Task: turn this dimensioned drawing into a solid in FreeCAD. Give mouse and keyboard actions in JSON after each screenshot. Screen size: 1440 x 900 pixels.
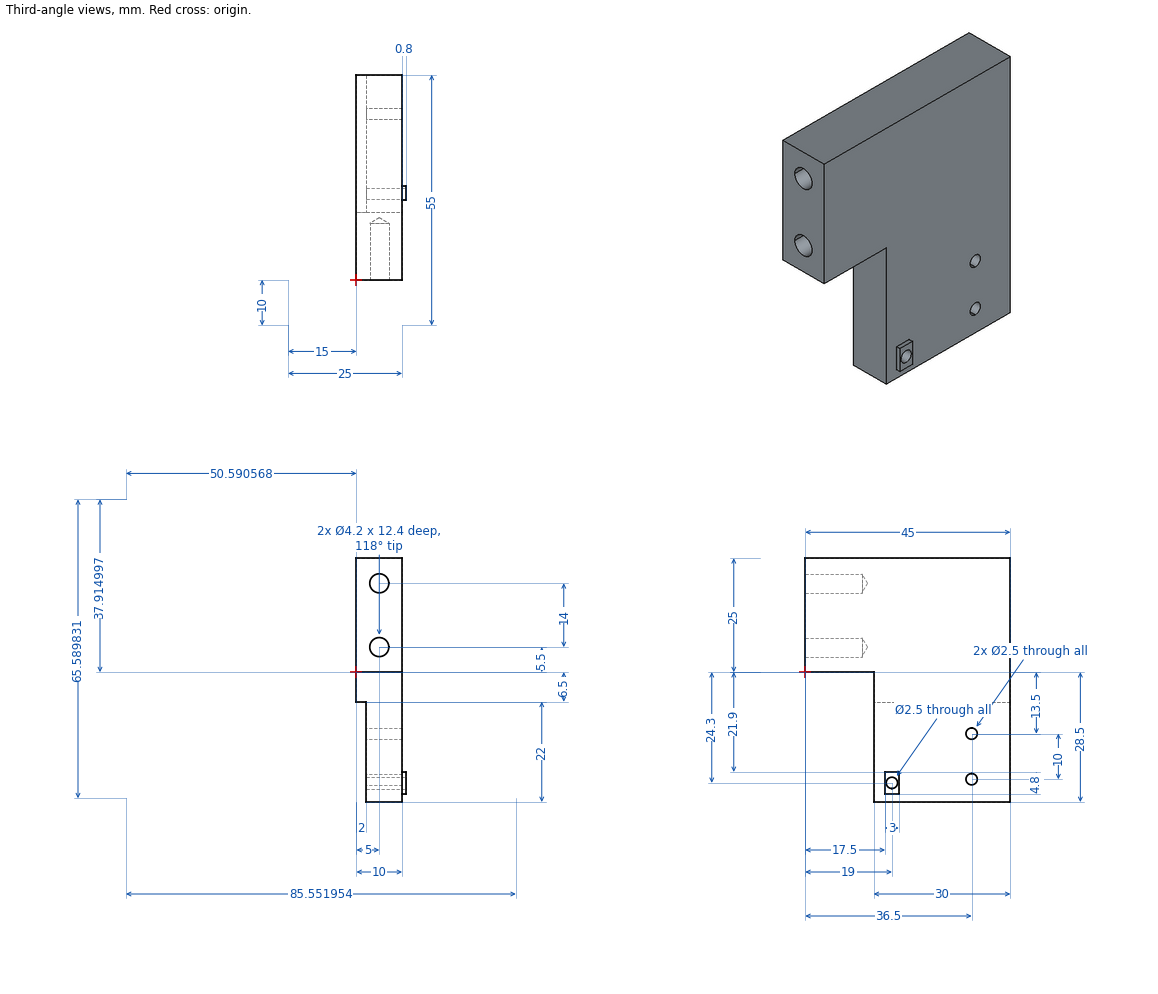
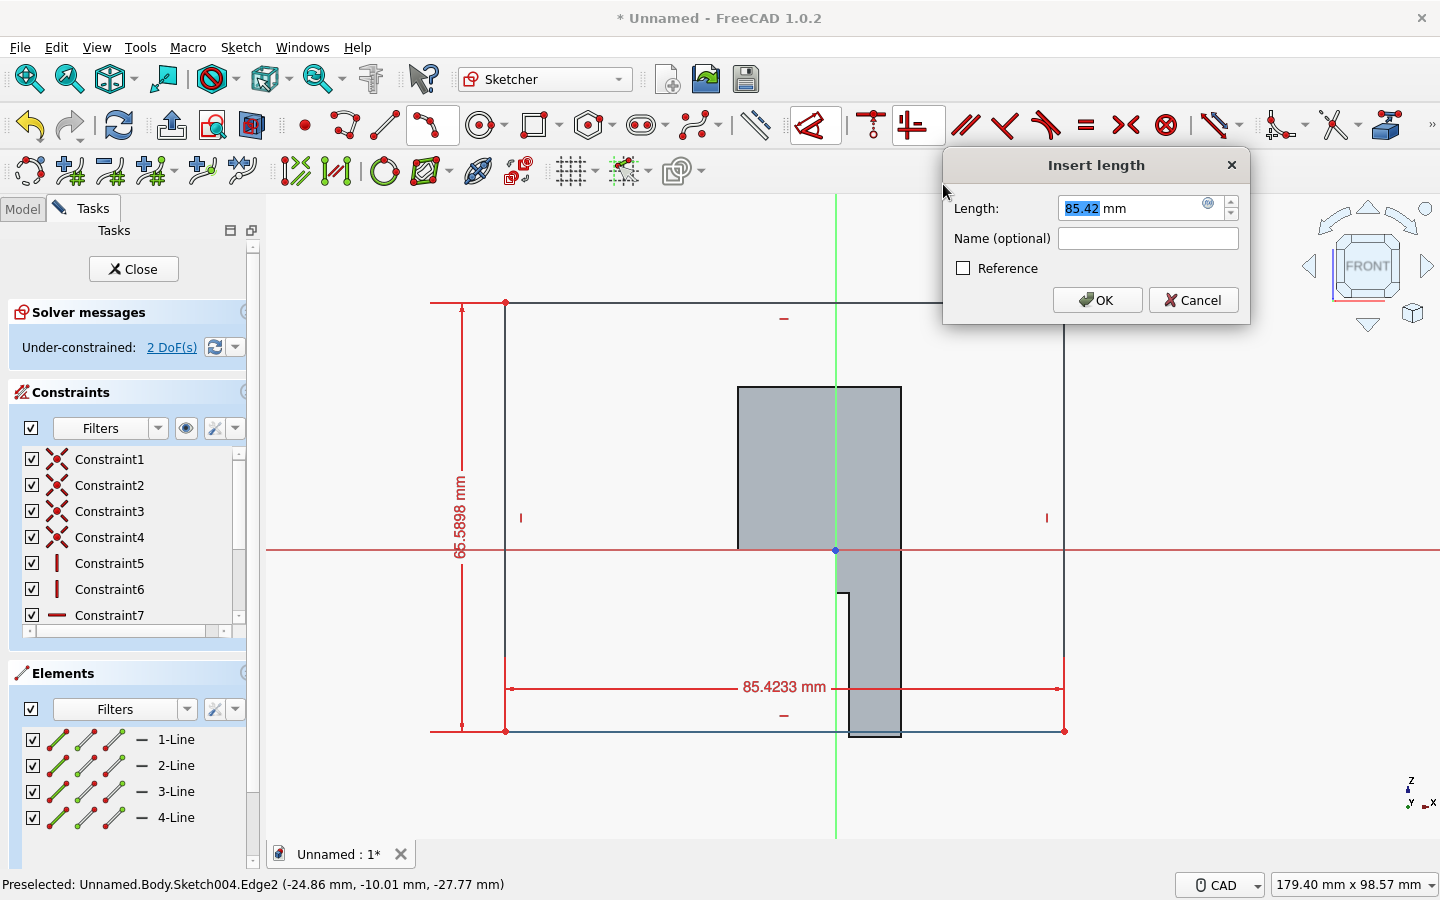
{"action": "type", "text": "85.551954"}
{"action": "key", "text": "Return"}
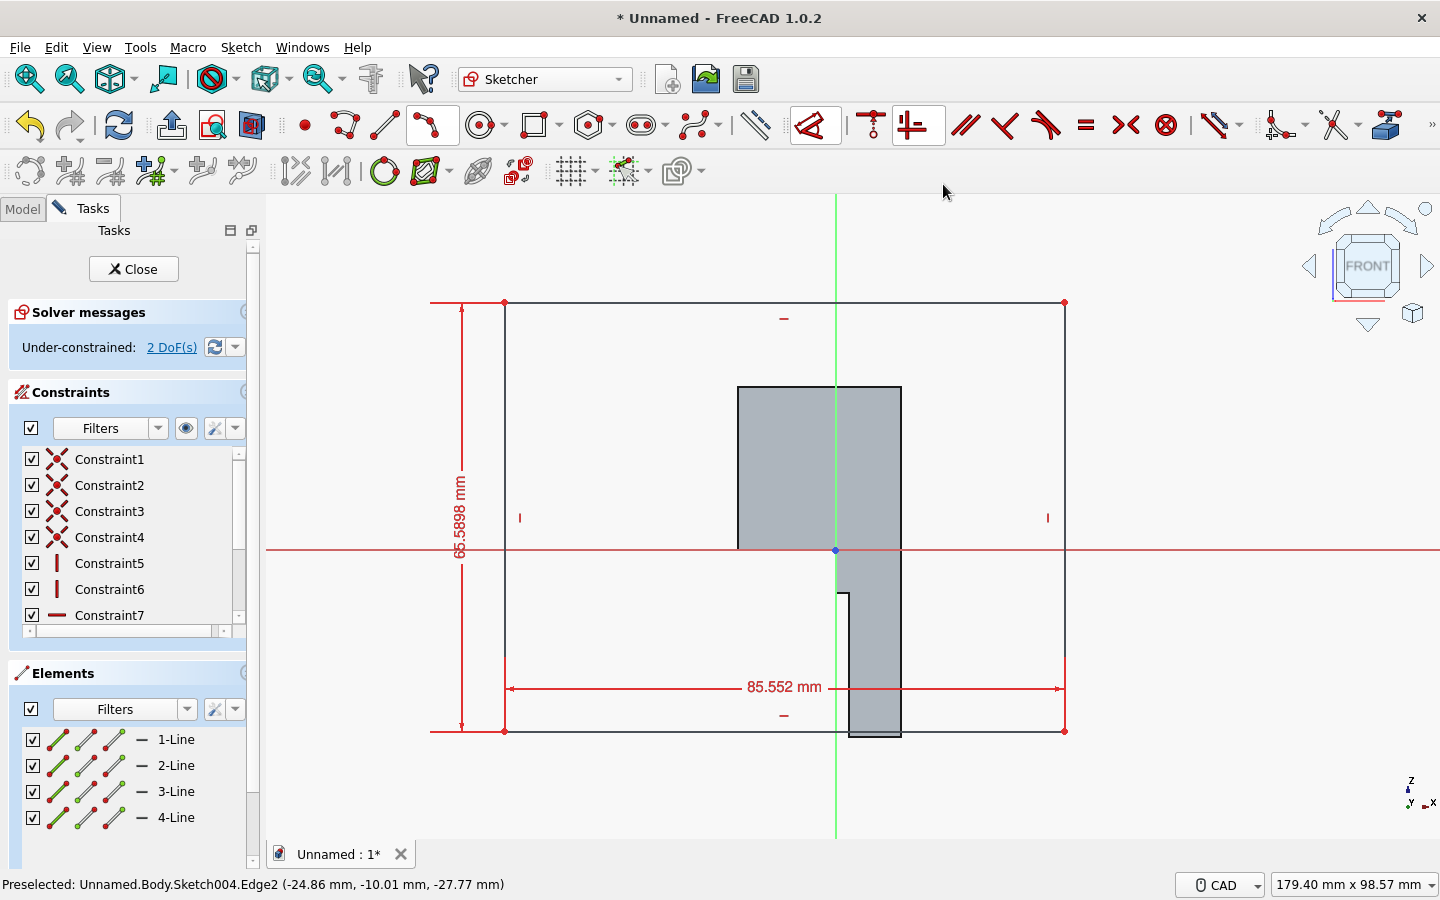
{"action": "left_click", "coordinate": [505, 303]}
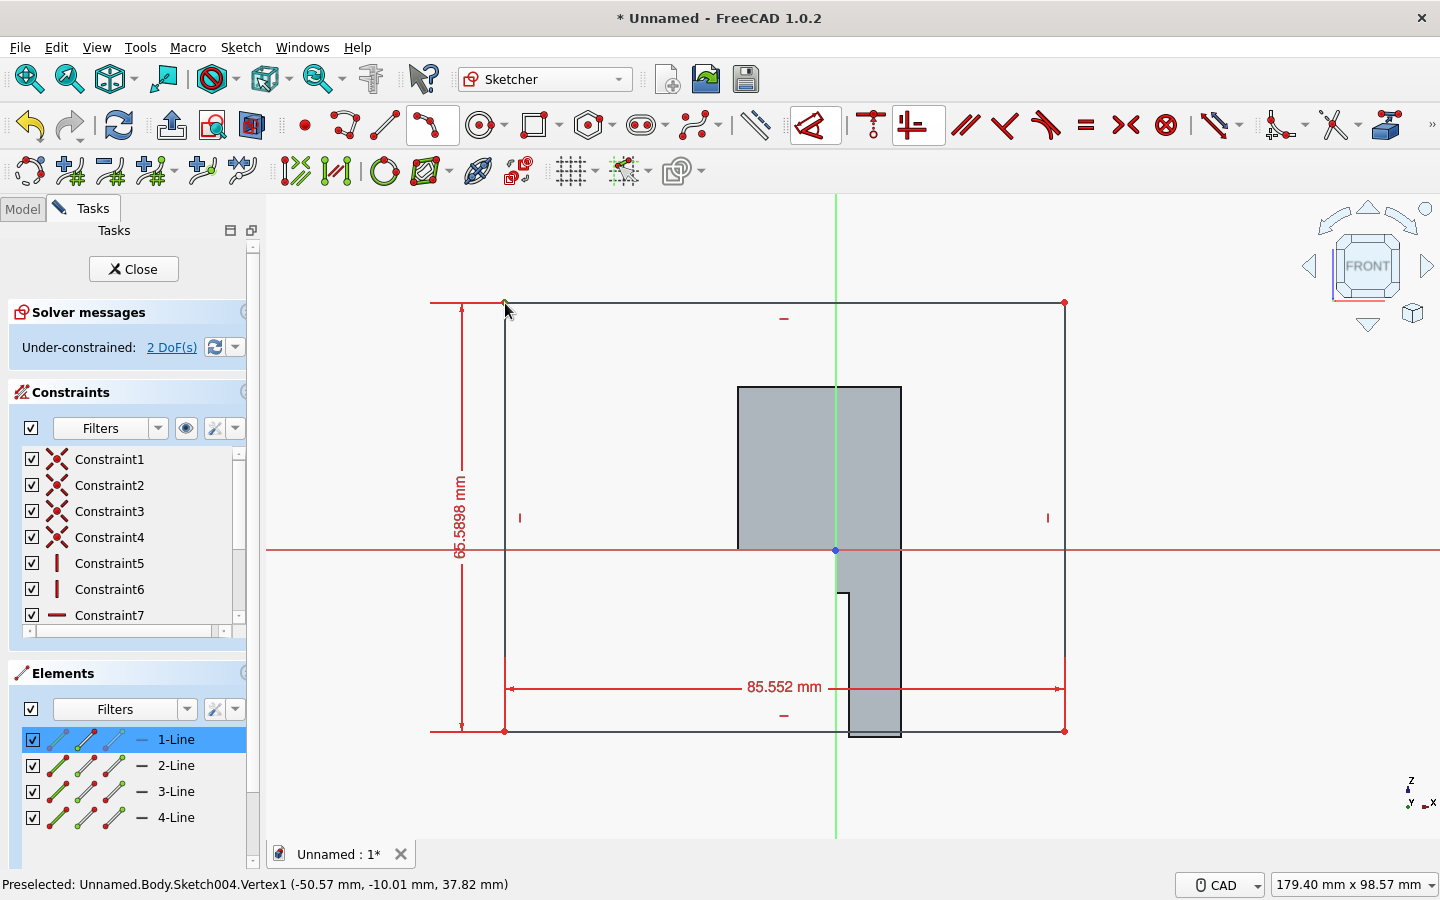
{"action": "left_click", "coordinate": [836, 126]}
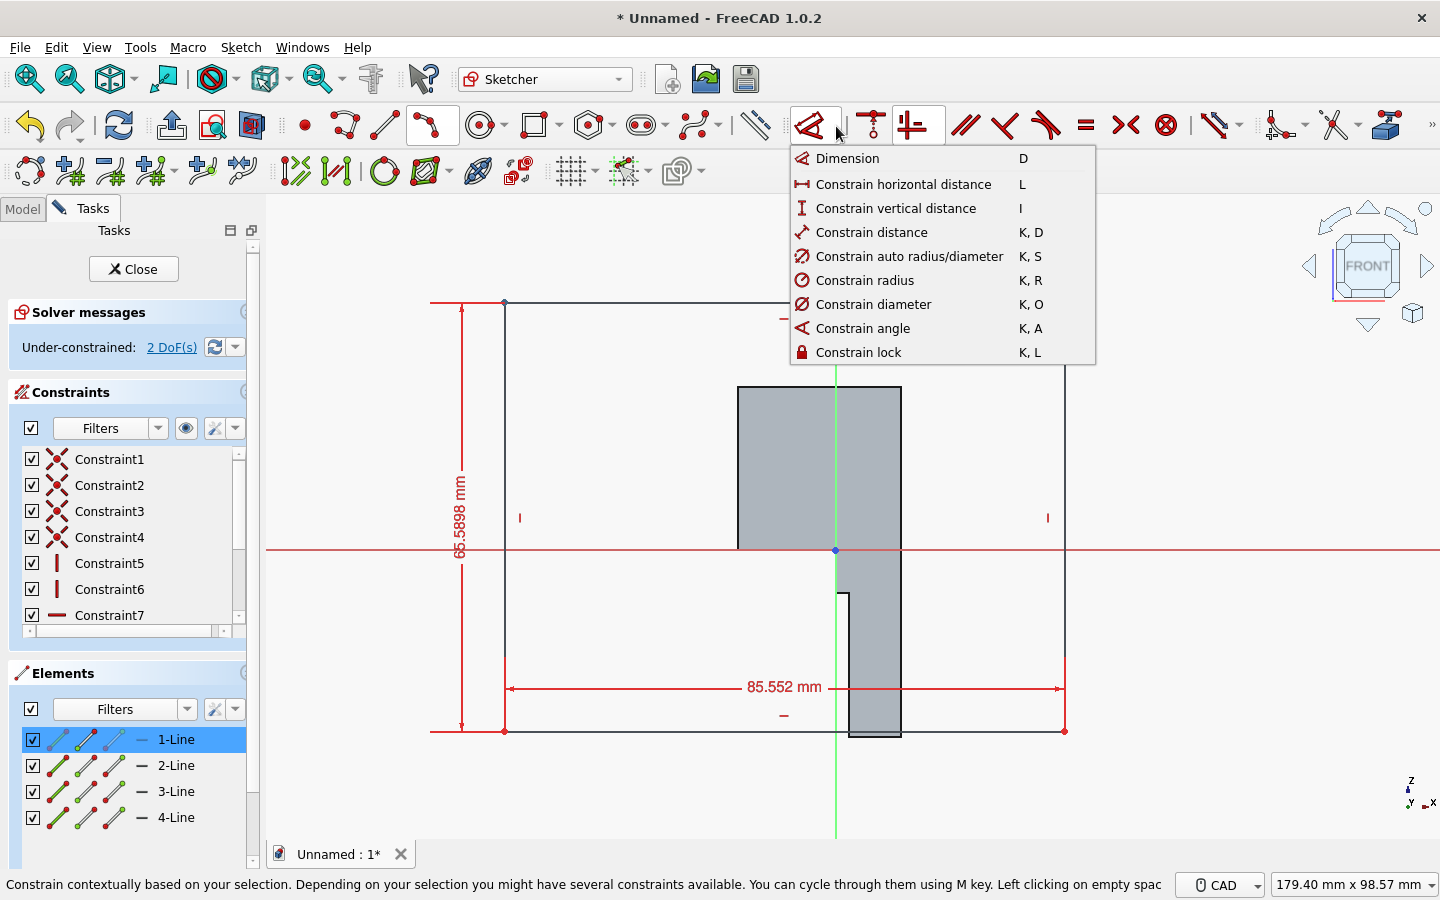
{"action": "left_click", "coordinate": [943, 184]}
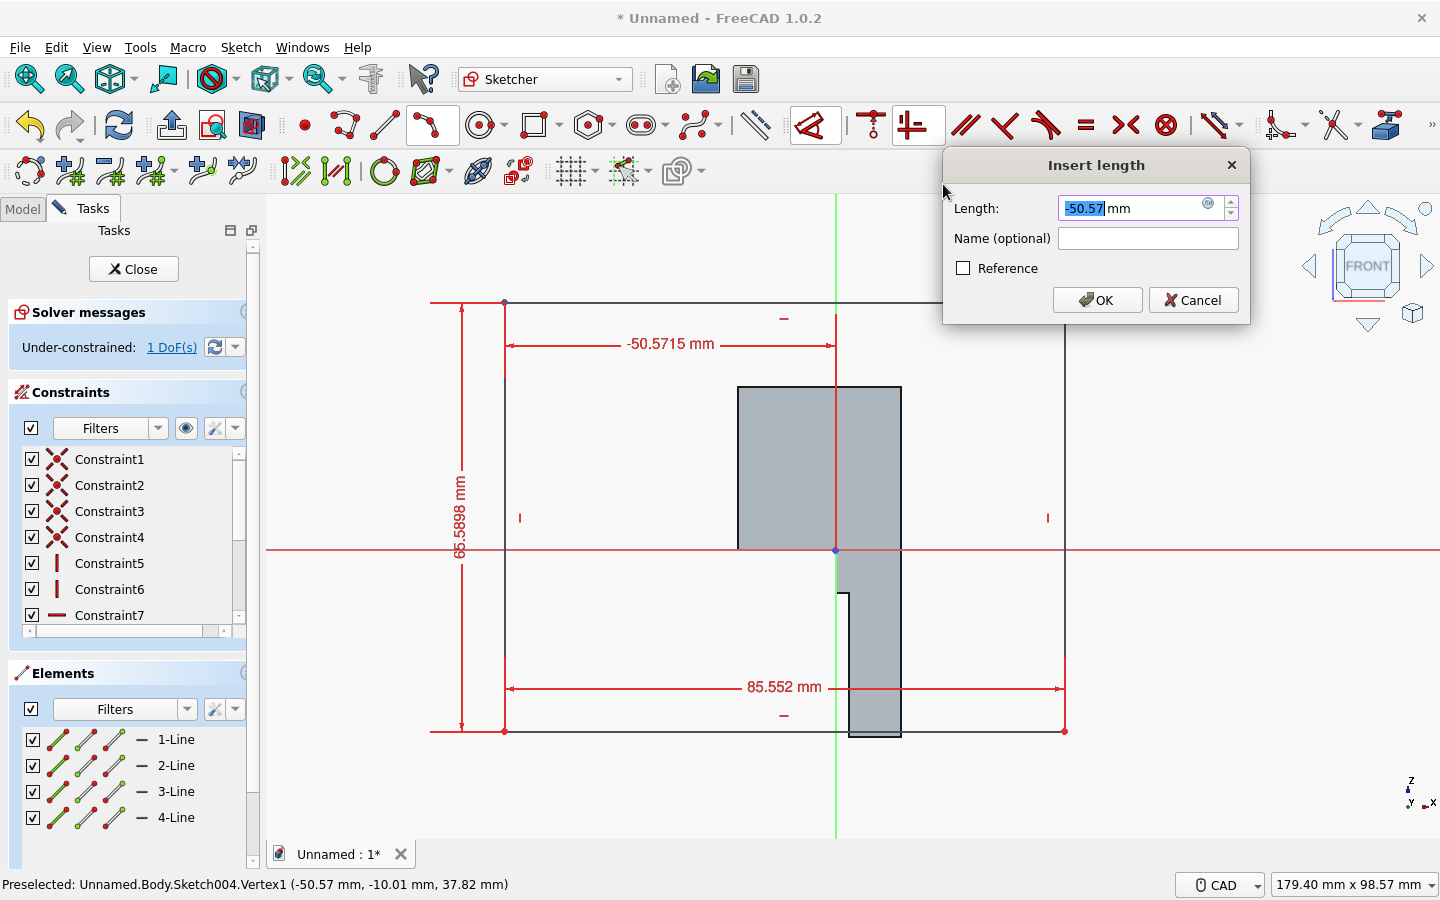
{"action": "type", "text": "-50.590568"}
{"action": "key", "text": "Return"}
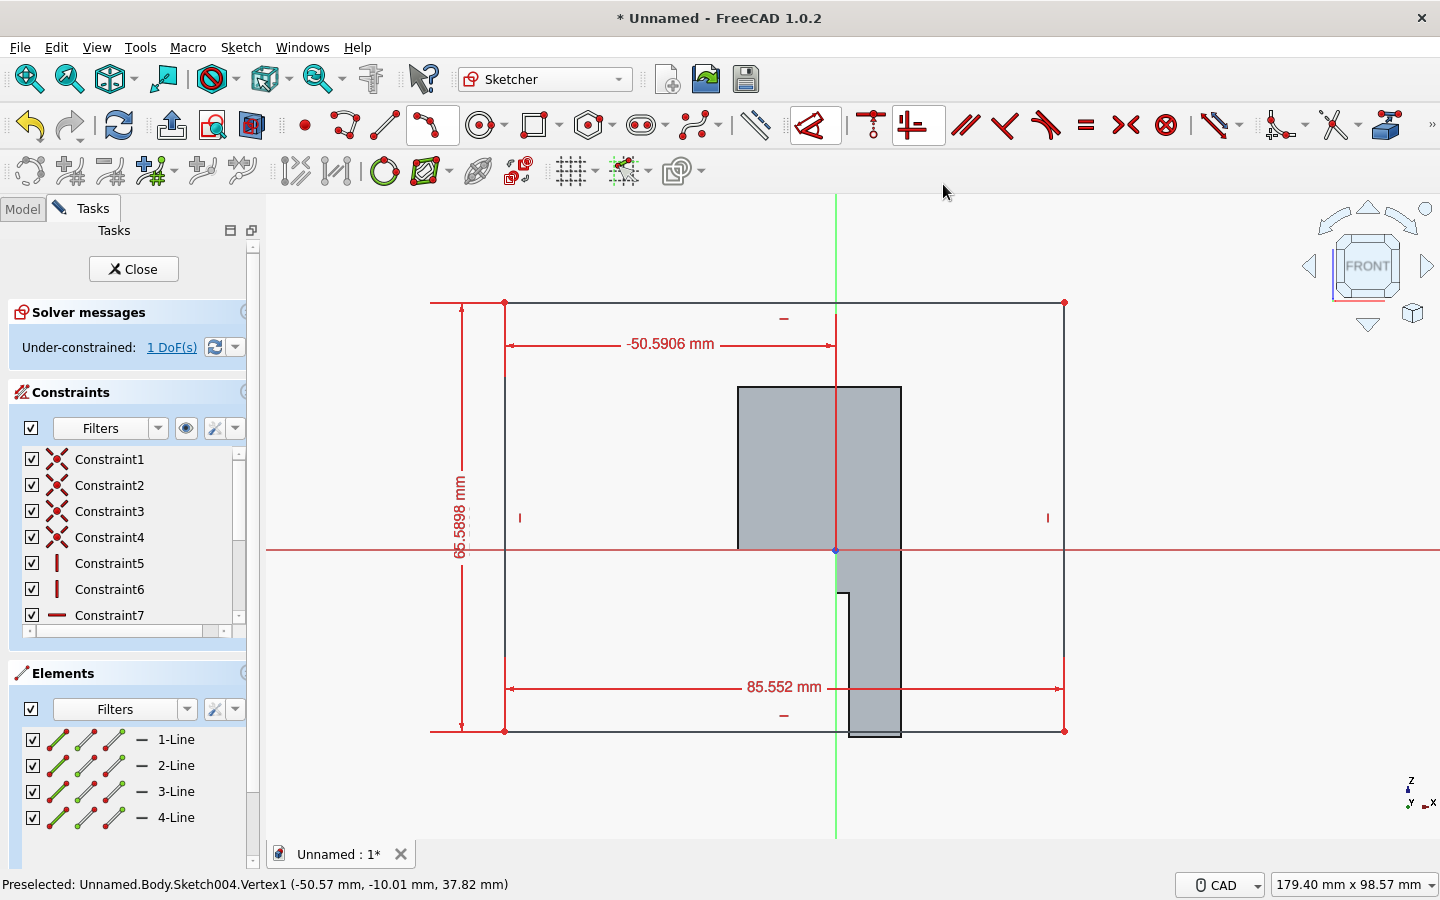
{"action": "left_click", "coordinate": [505, 303]}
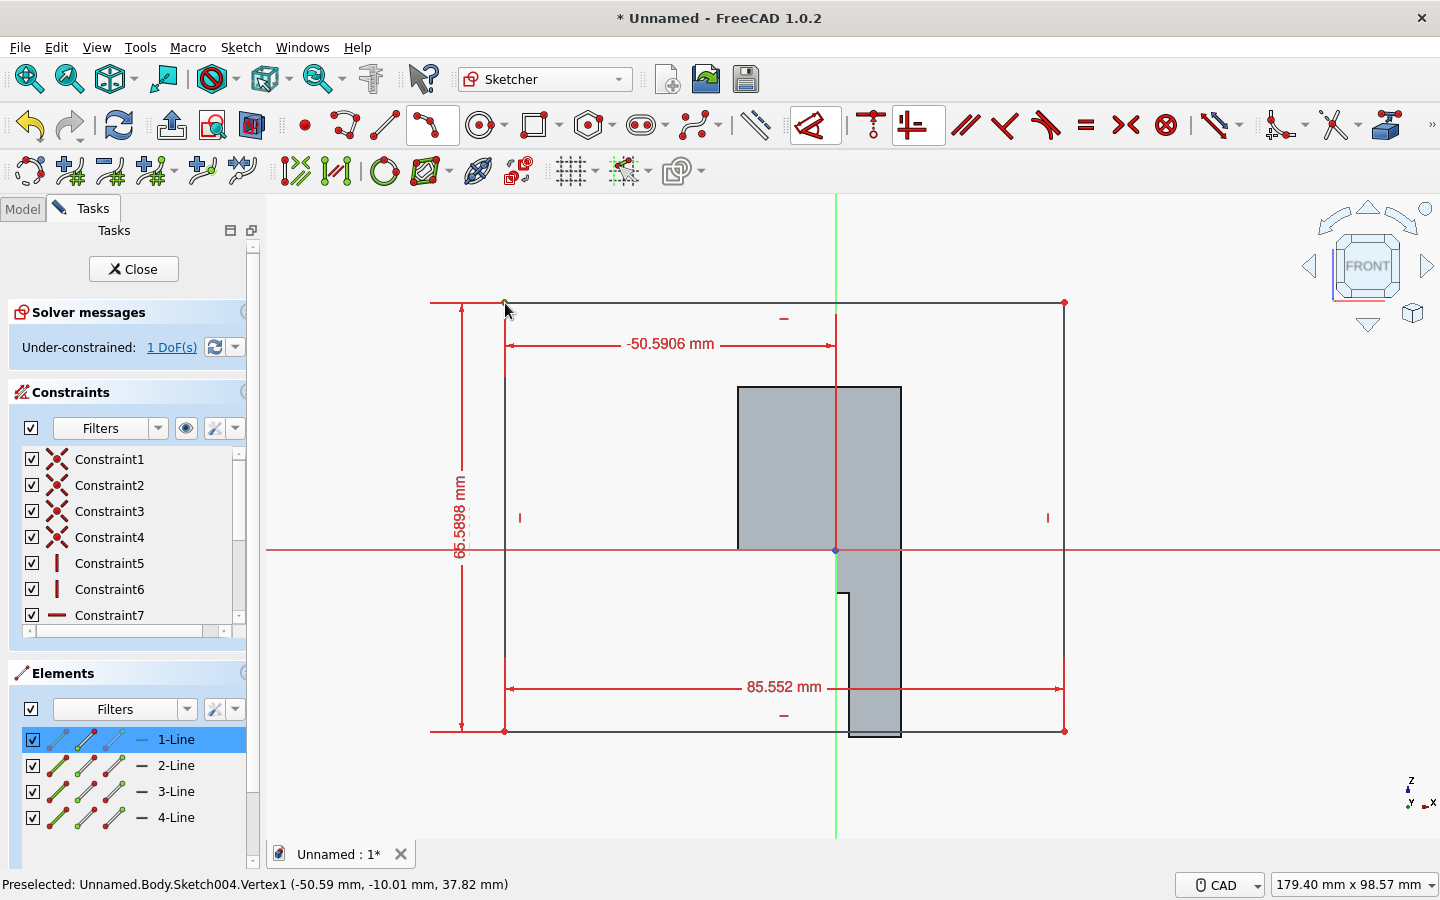
{"action": "left_click", "coordinate": [836, 126]}